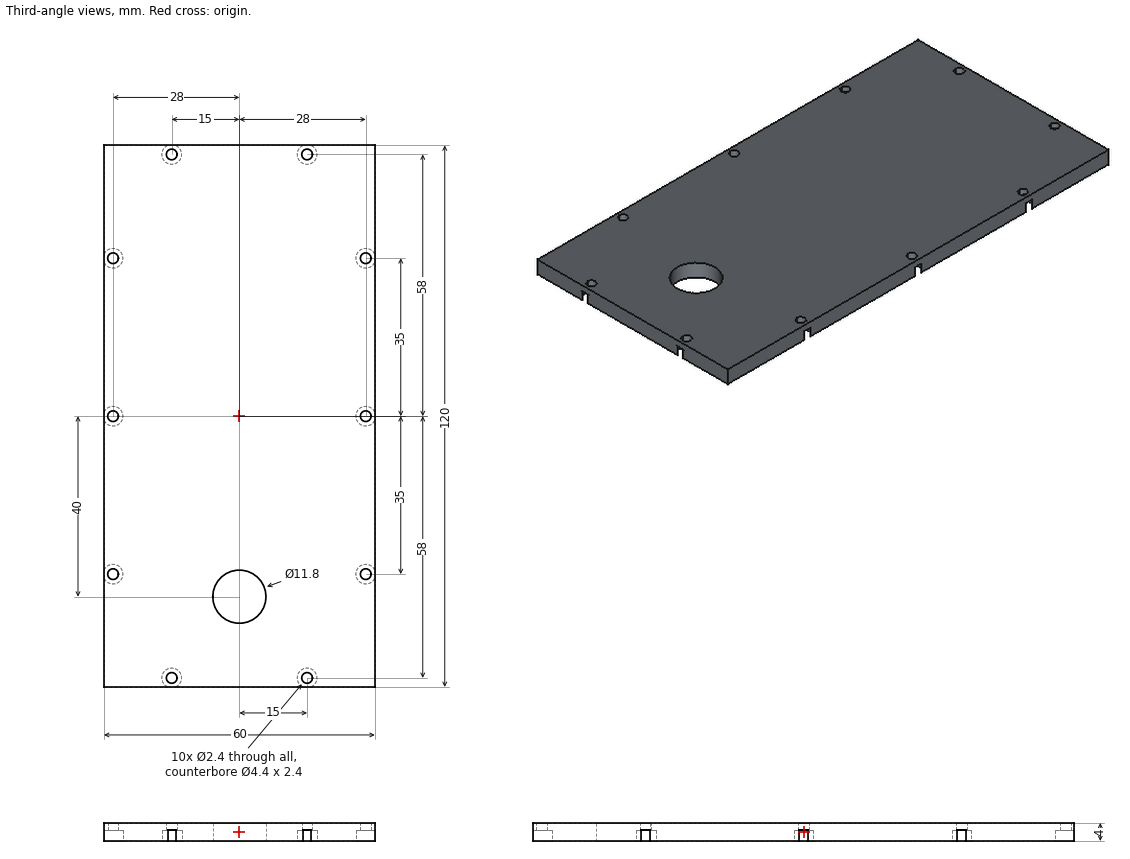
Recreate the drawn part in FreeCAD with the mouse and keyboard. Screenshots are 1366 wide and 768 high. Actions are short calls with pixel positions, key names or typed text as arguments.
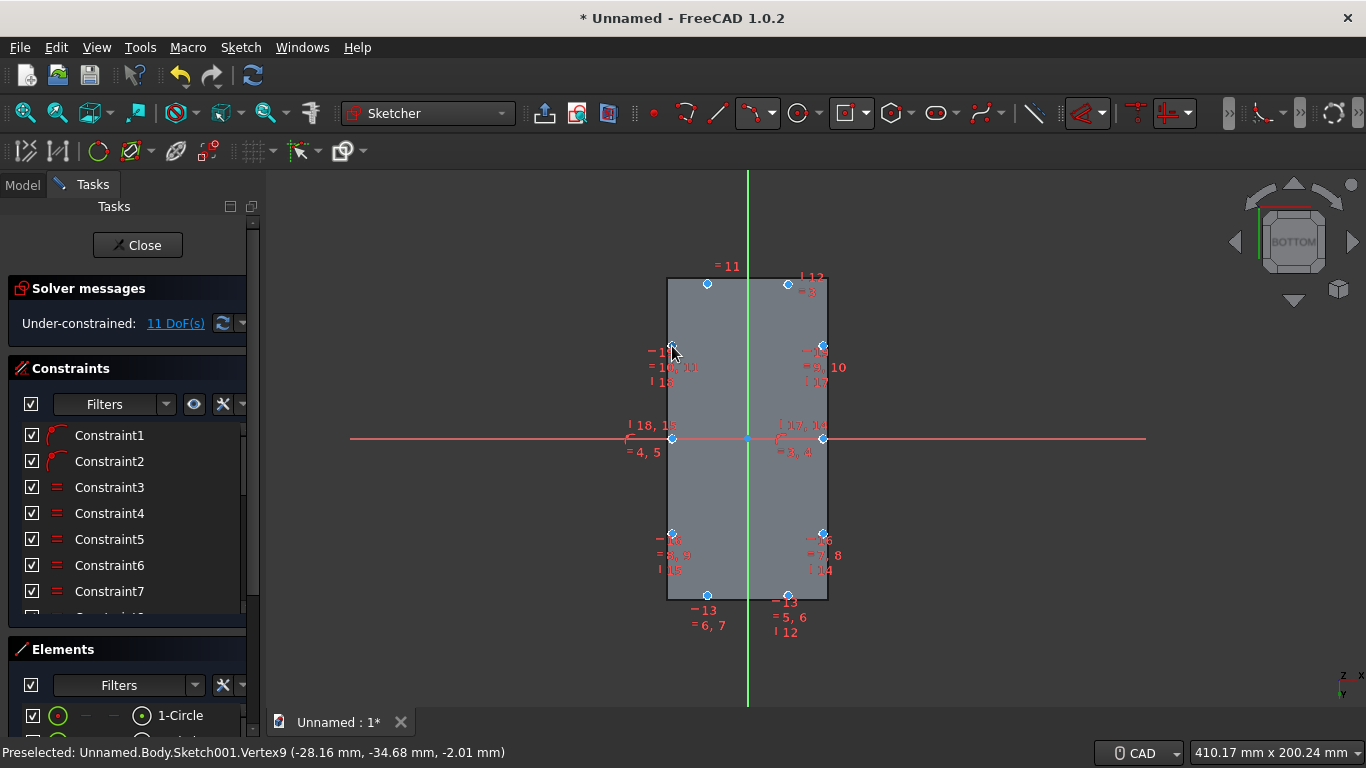
click(788, 284)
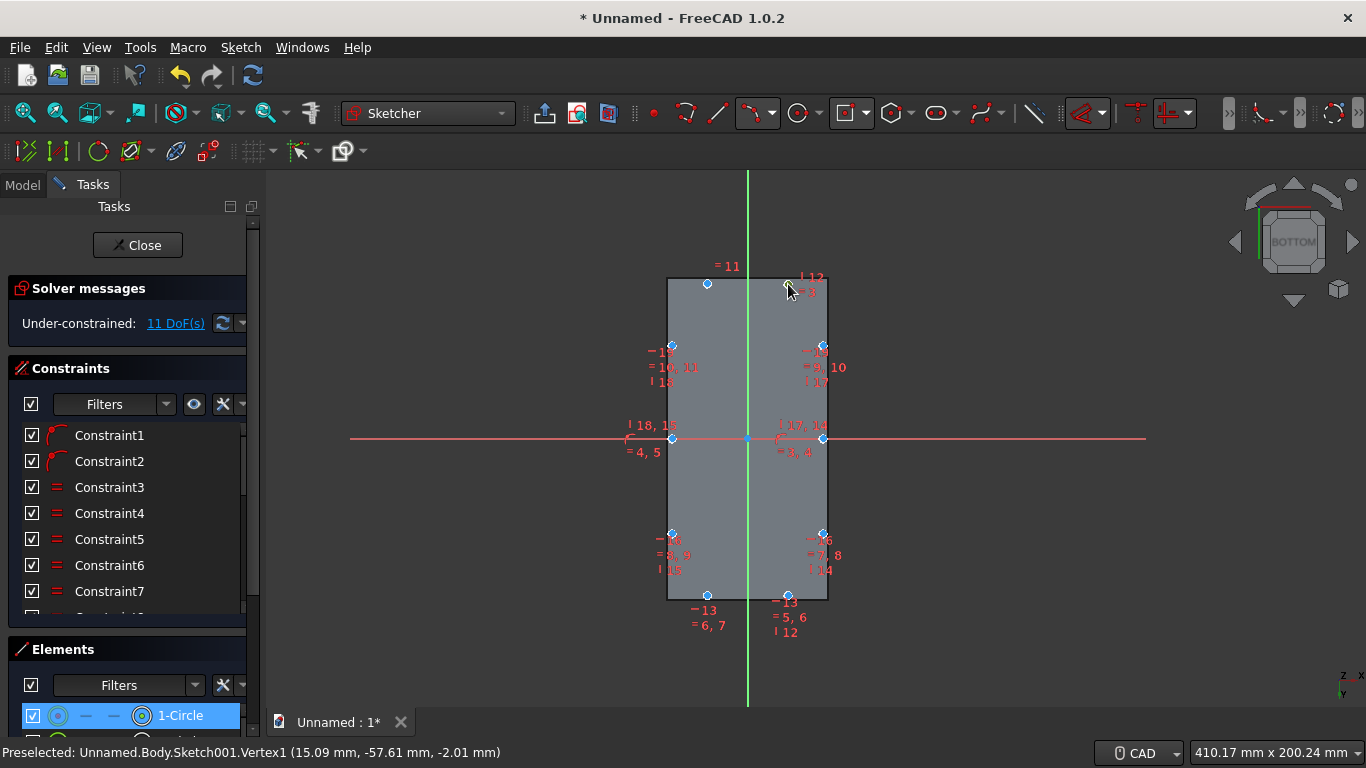
click(707, 284)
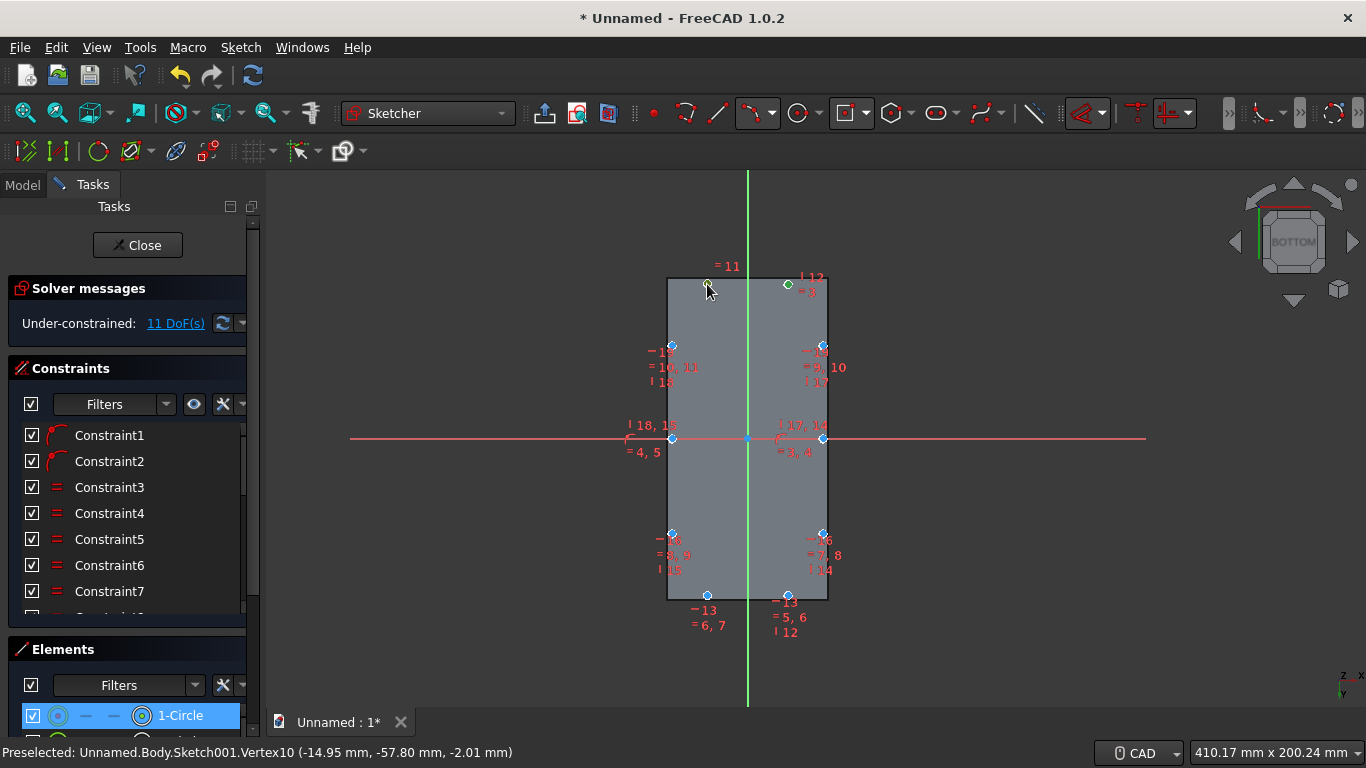
click(1190, 114)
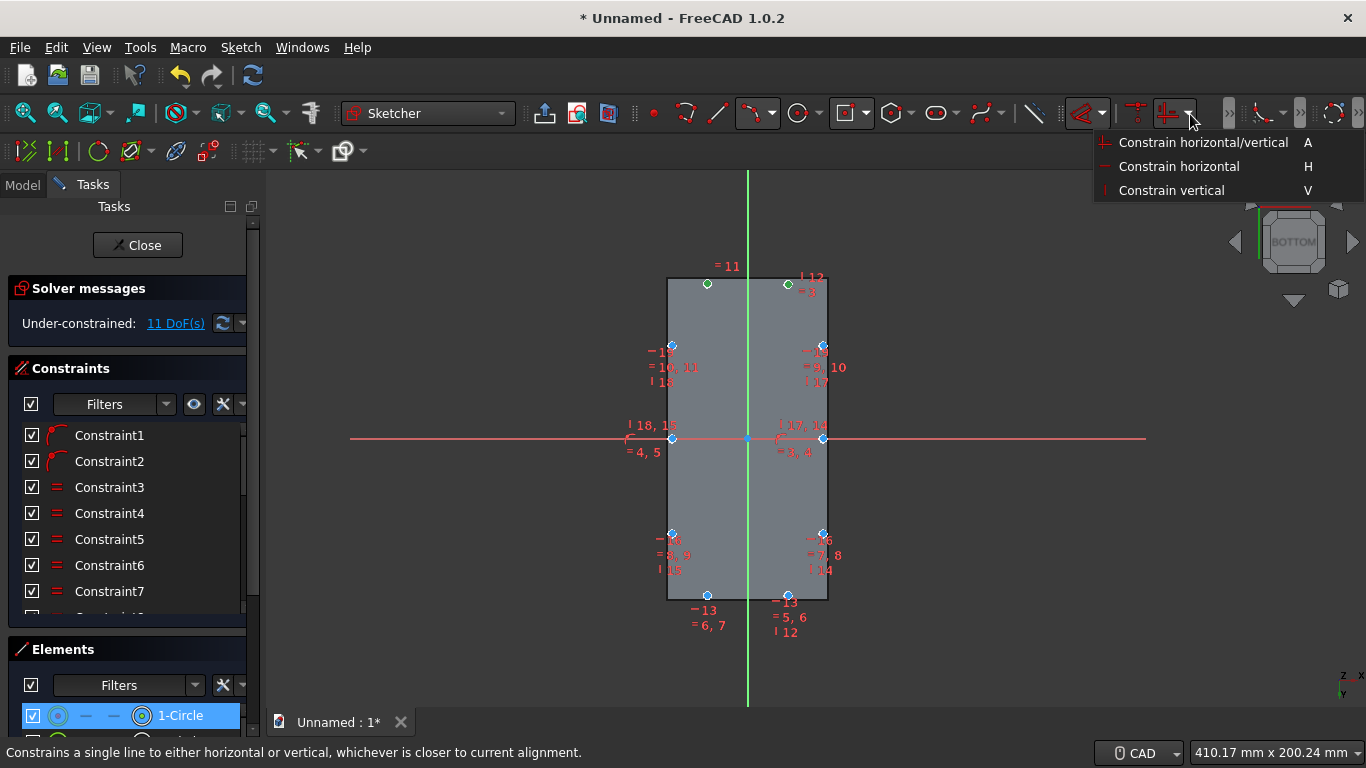
click(1229, 166)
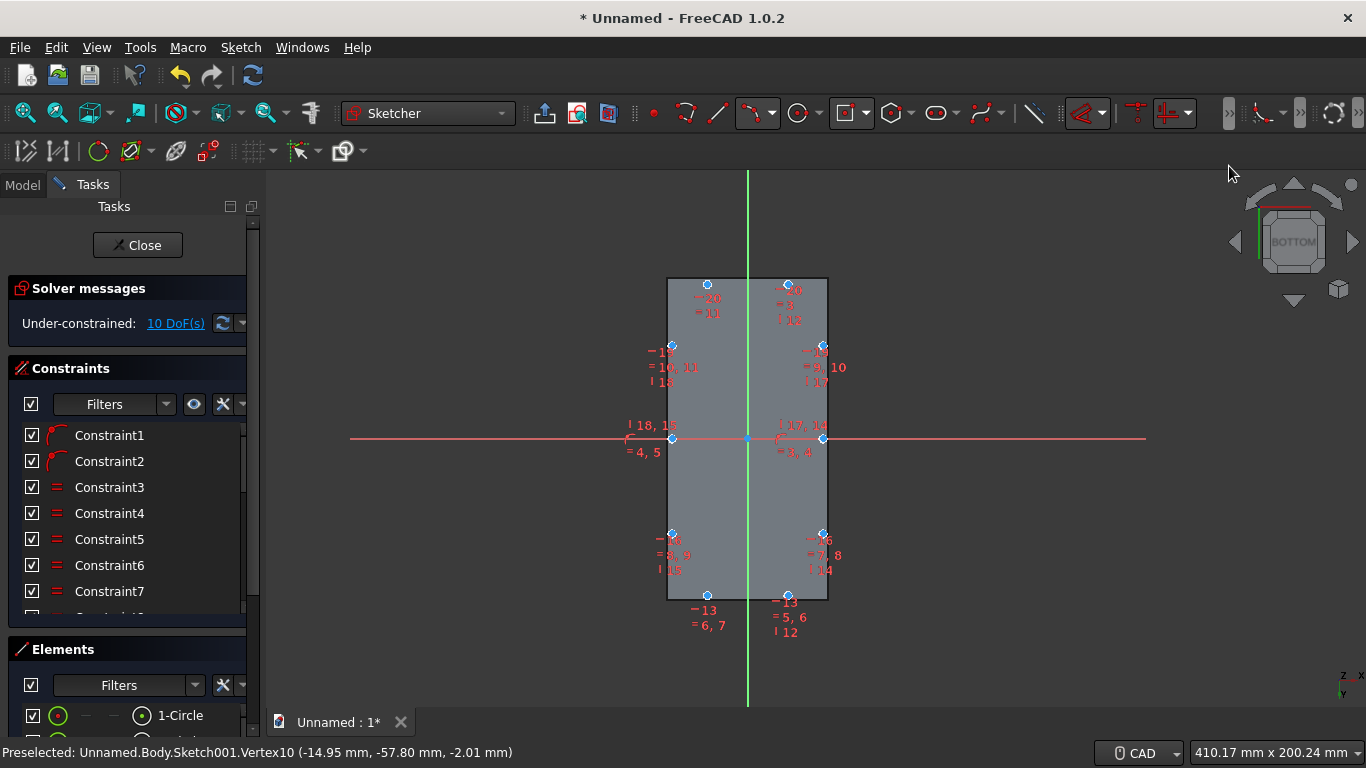
scroll(791, 282, up, 10)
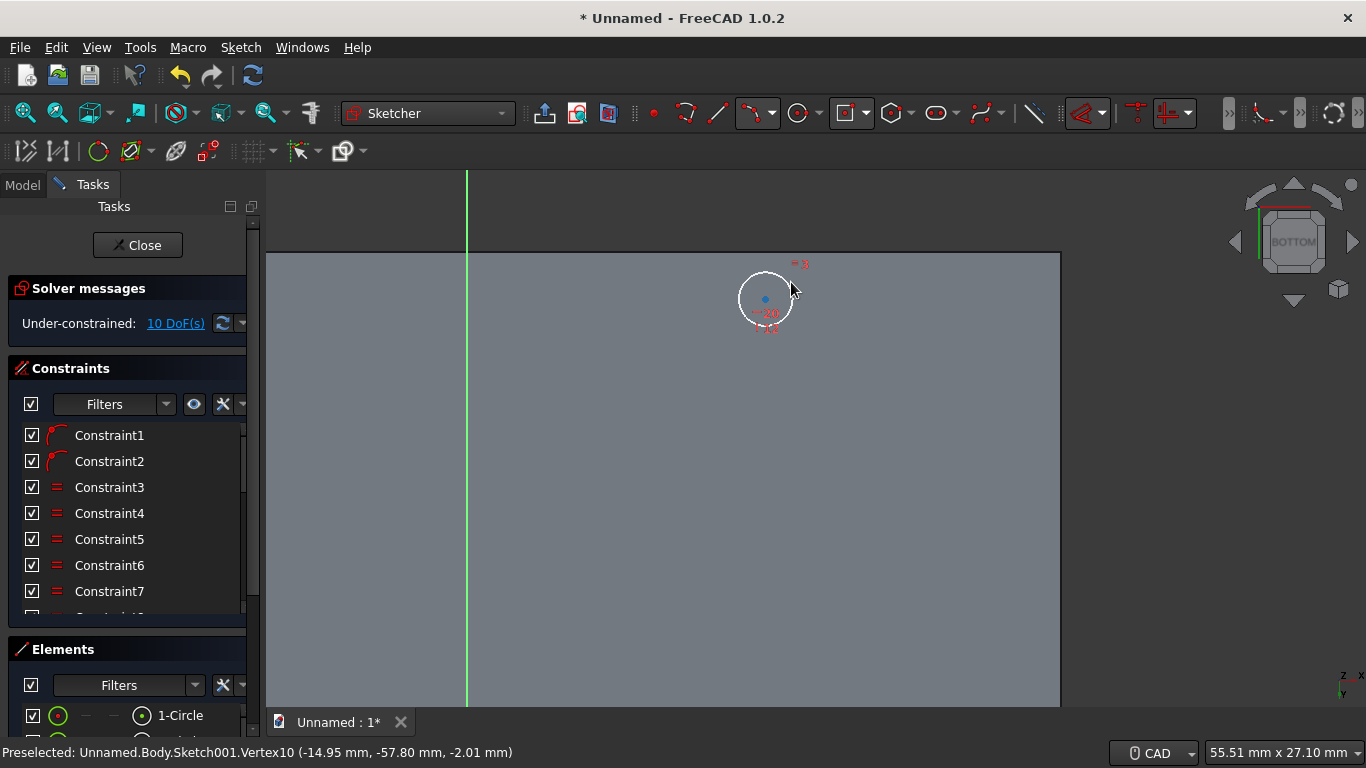
click(785, 280)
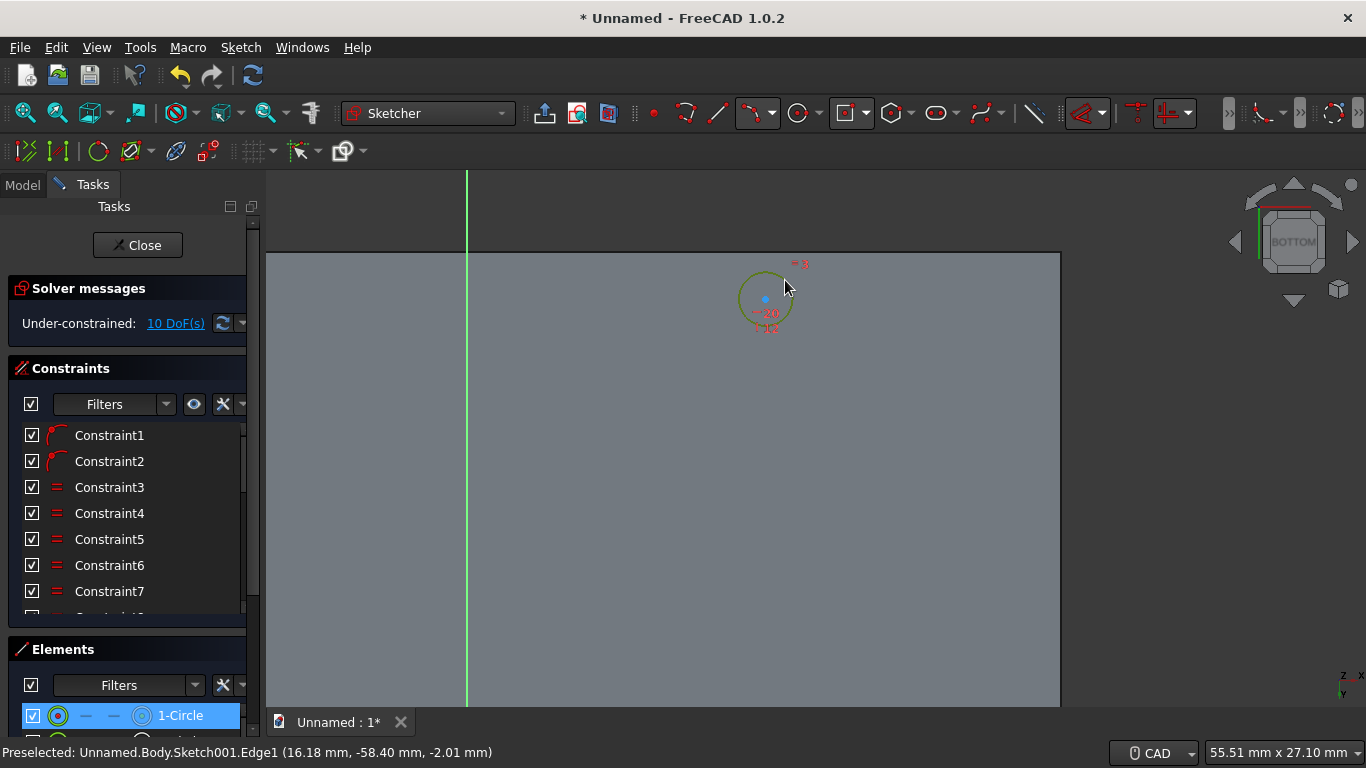
click(1104, 114)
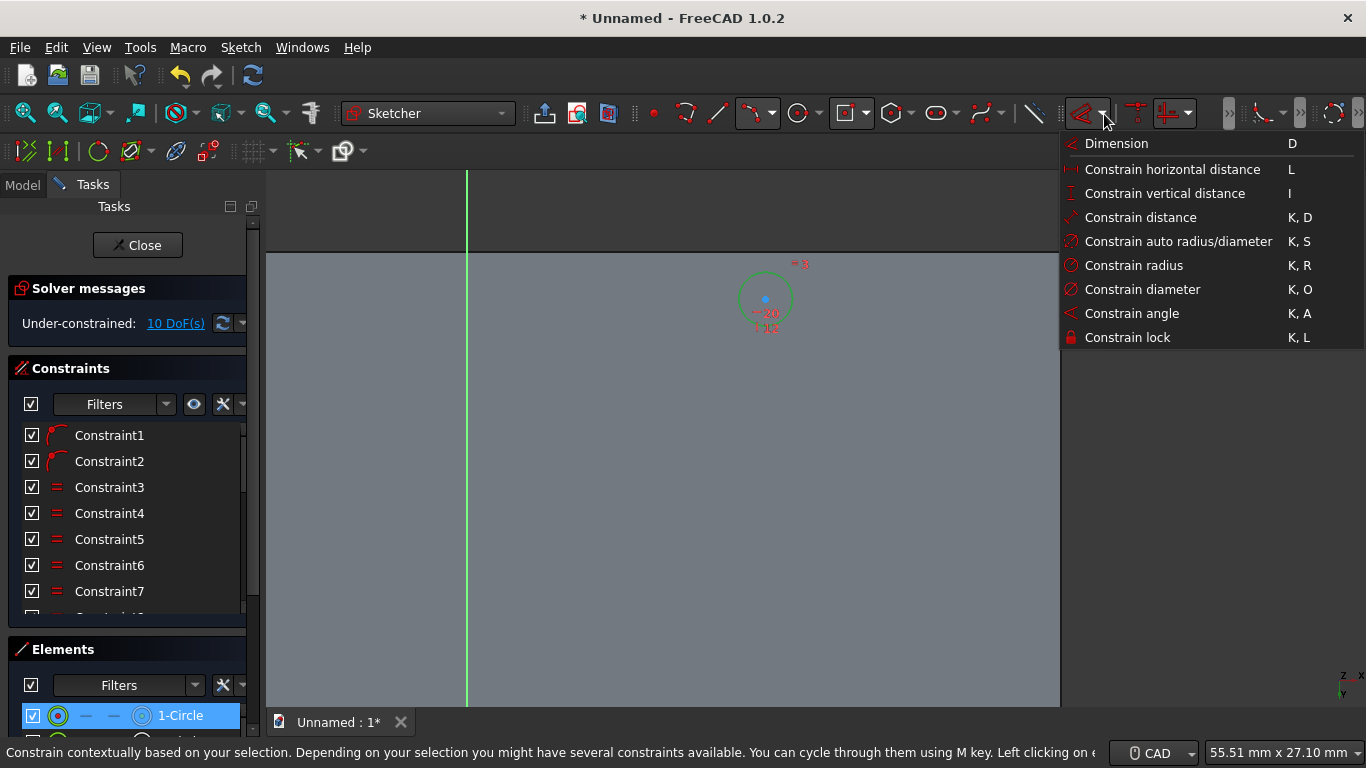
click(1212, 289)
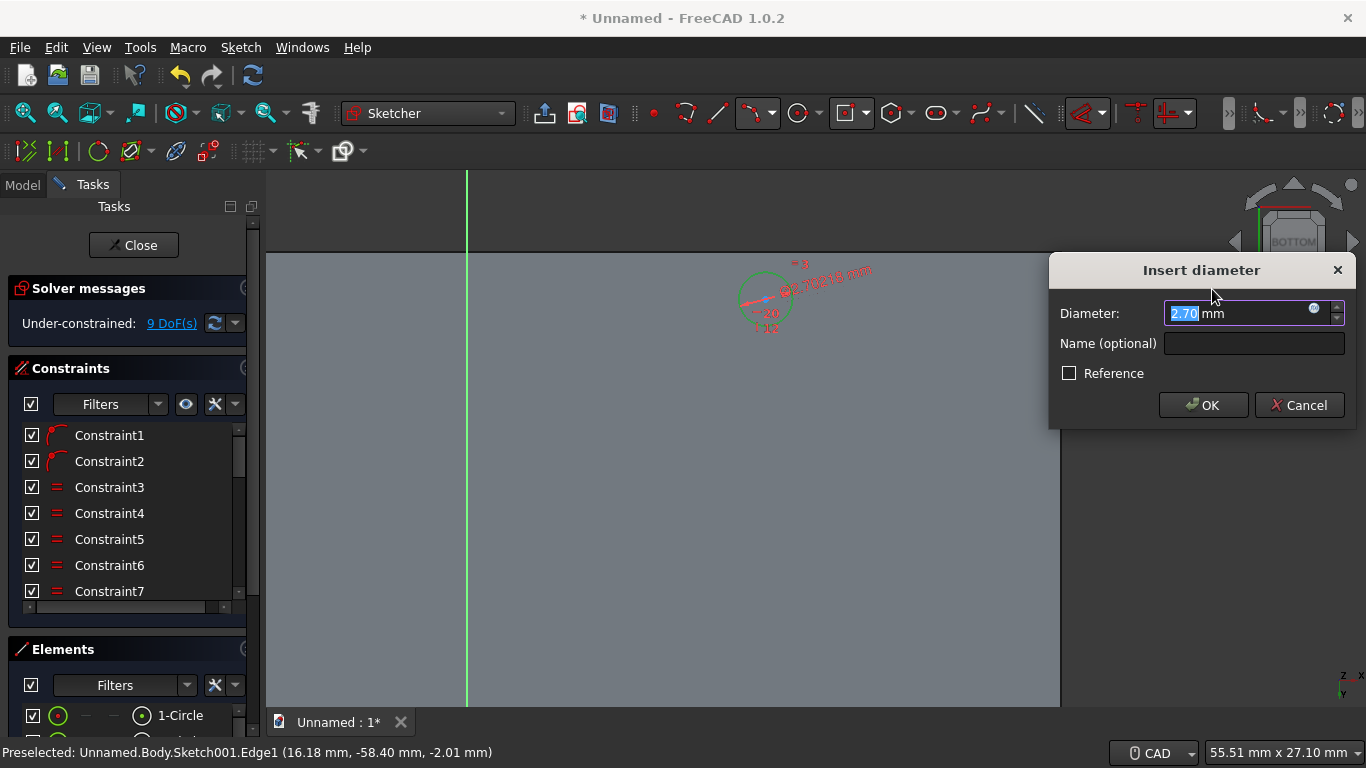
text(2.4)
key(Return)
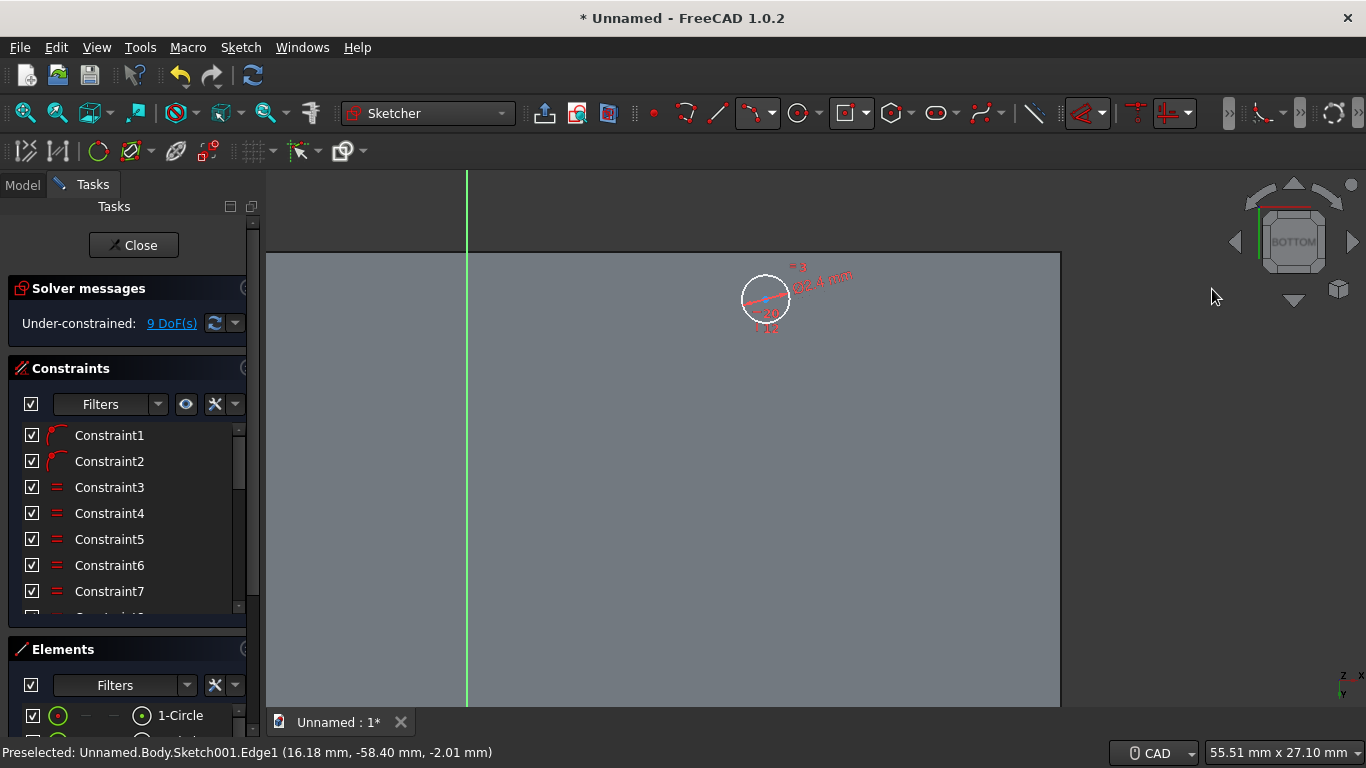
scroll(791, 282, down, 10)